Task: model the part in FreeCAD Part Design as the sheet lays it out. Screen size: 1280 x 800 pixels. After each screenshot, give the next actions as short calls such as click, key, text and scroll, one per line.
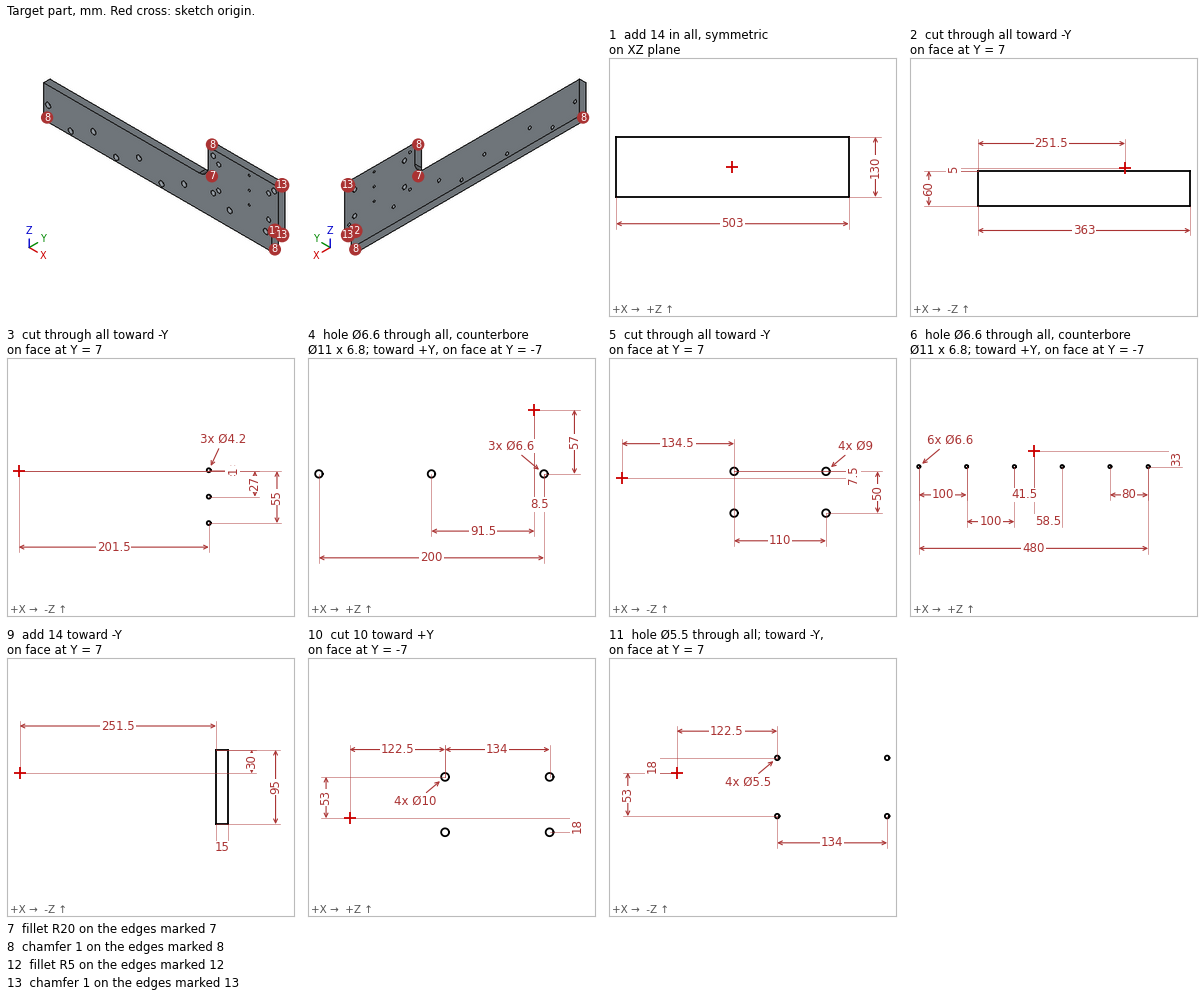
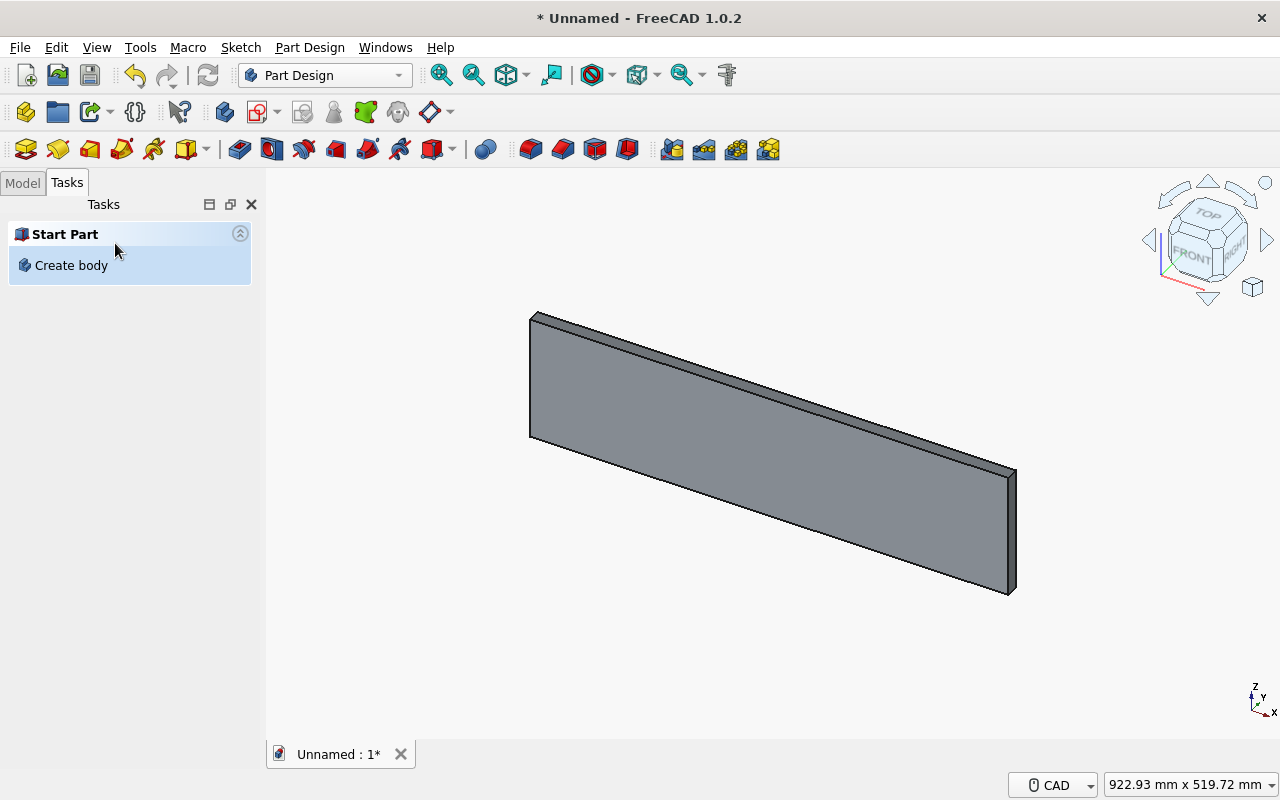
key(4)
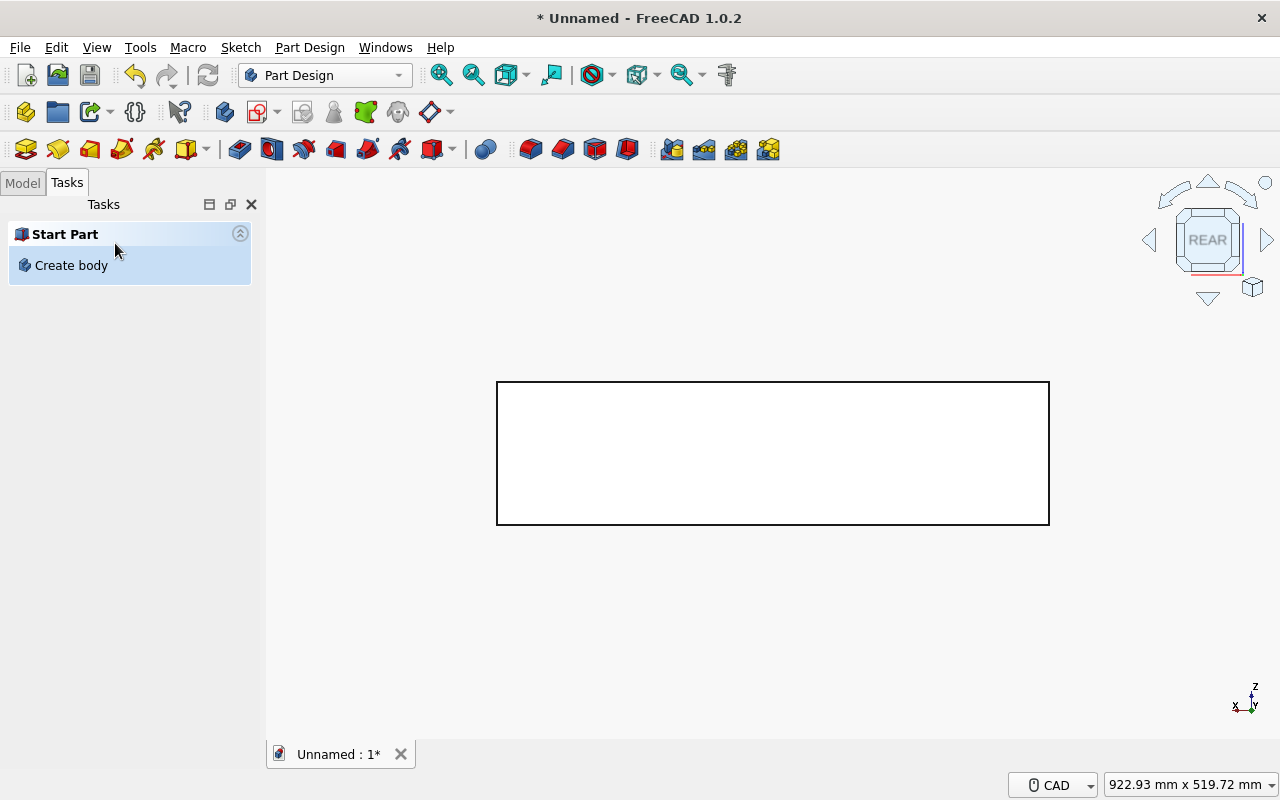
click(615, 452)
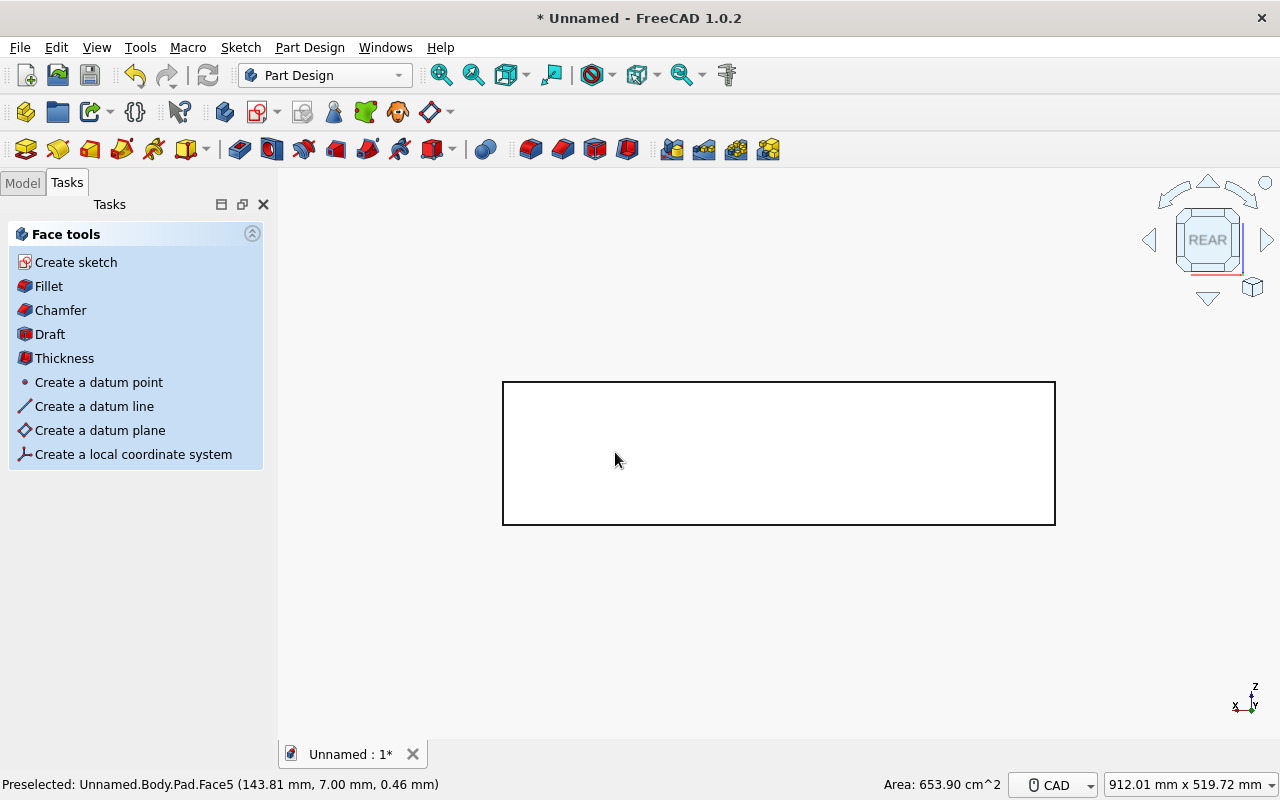
click(258, 112)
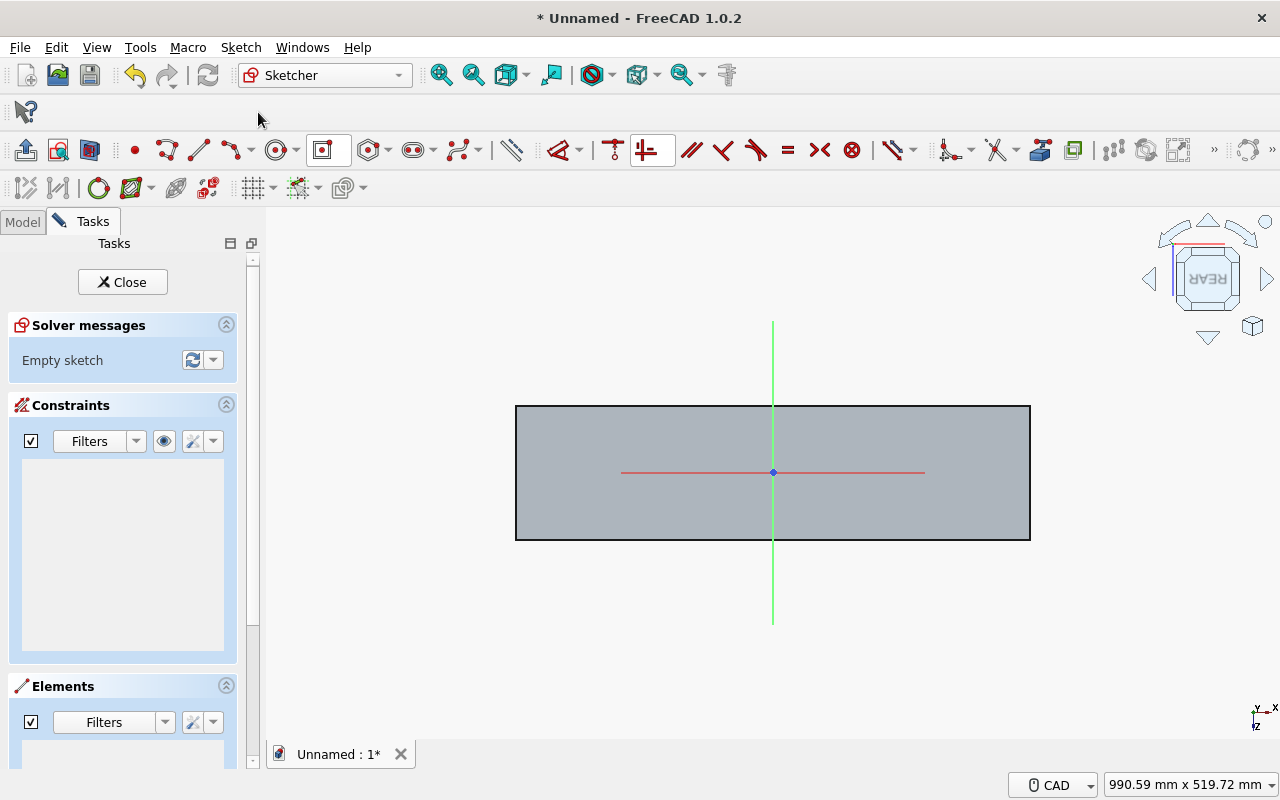
scroll(695, 574, up, 2)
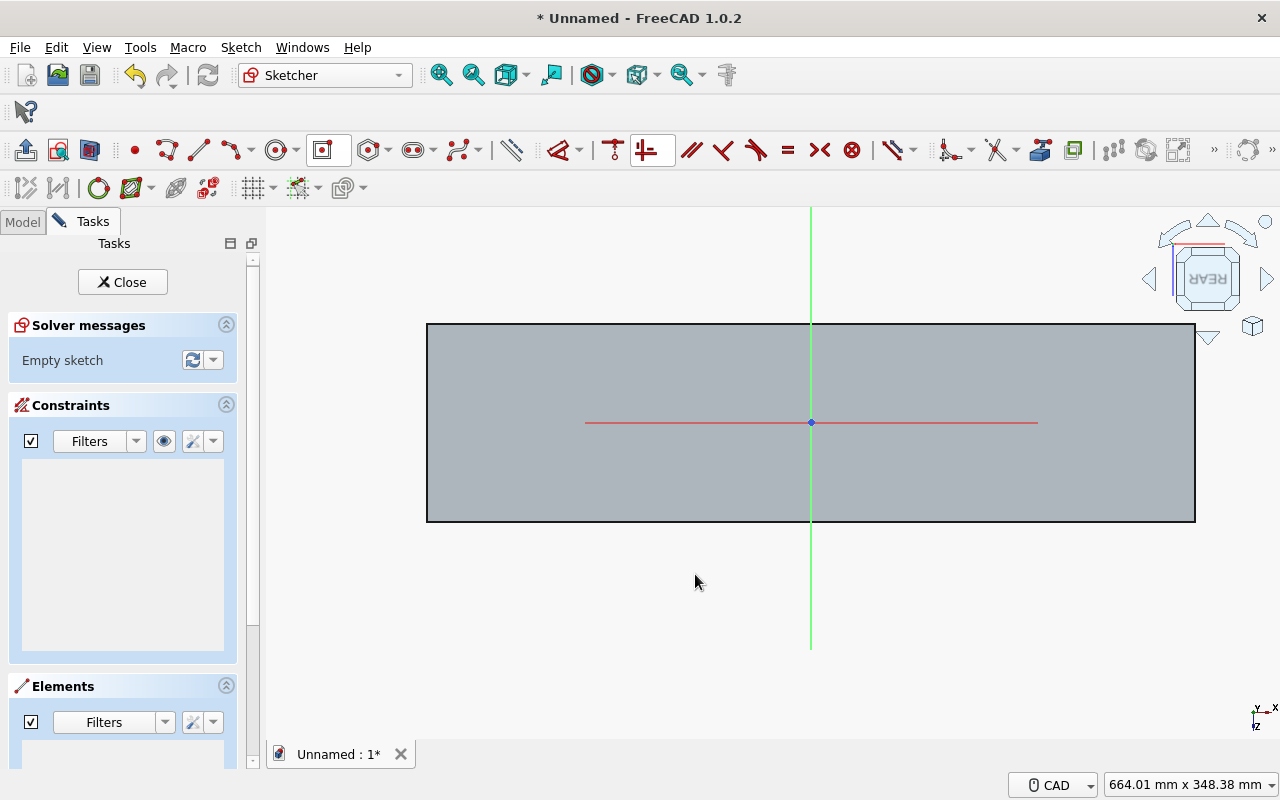
key(g)
key(r)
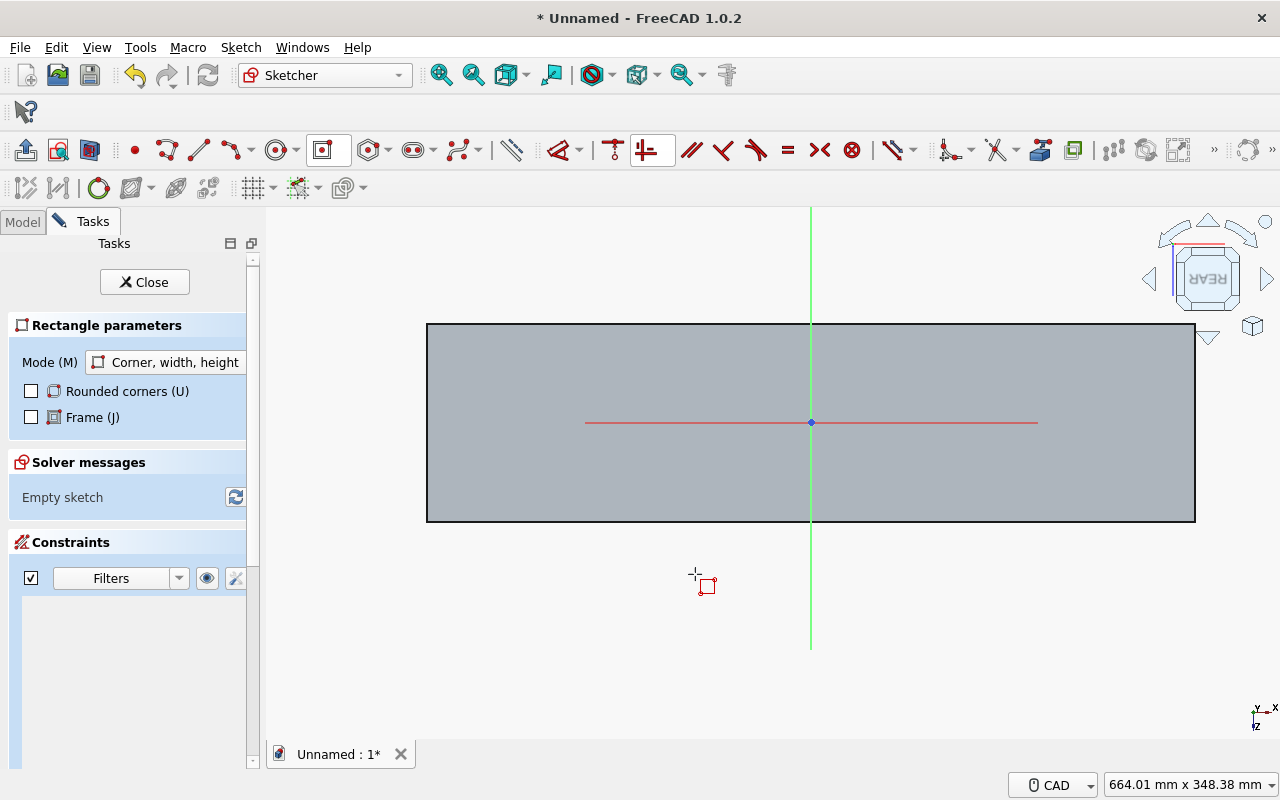
scroll(427, 431, up, 4)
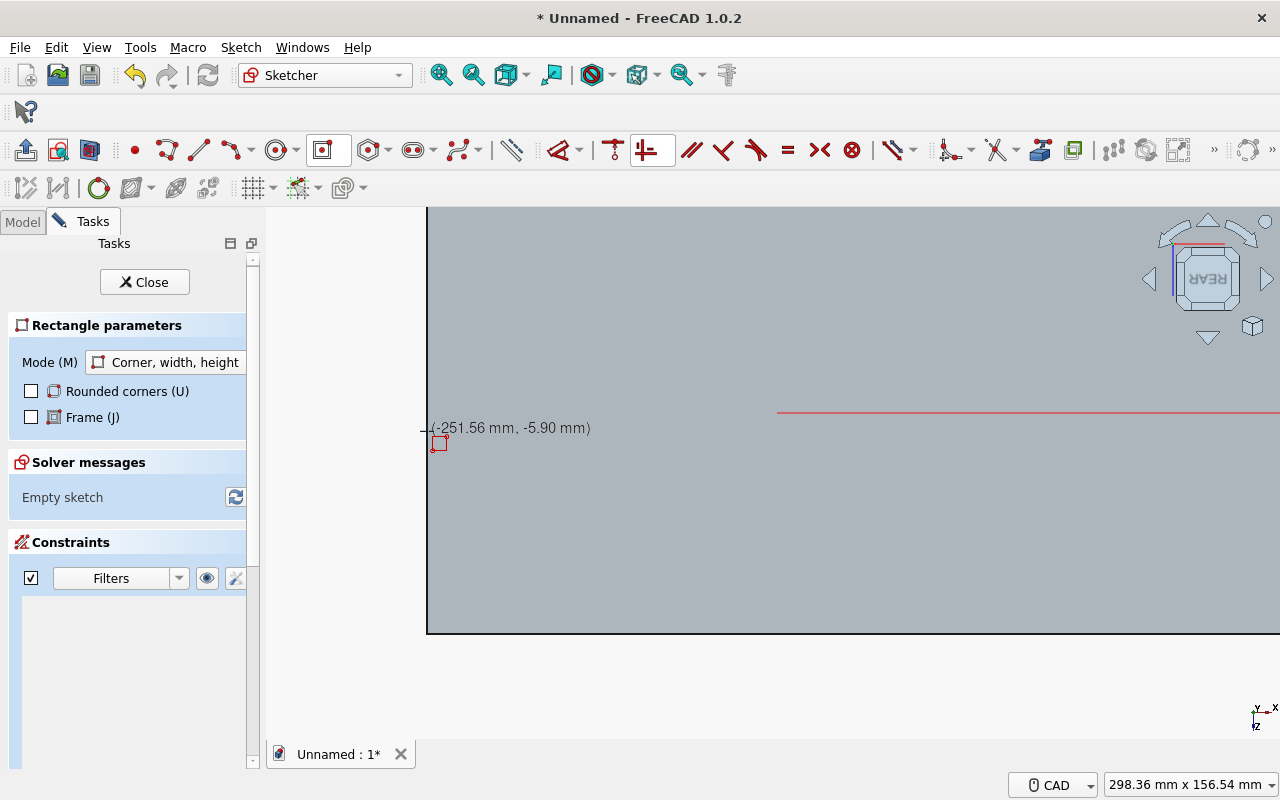
click(427, 430)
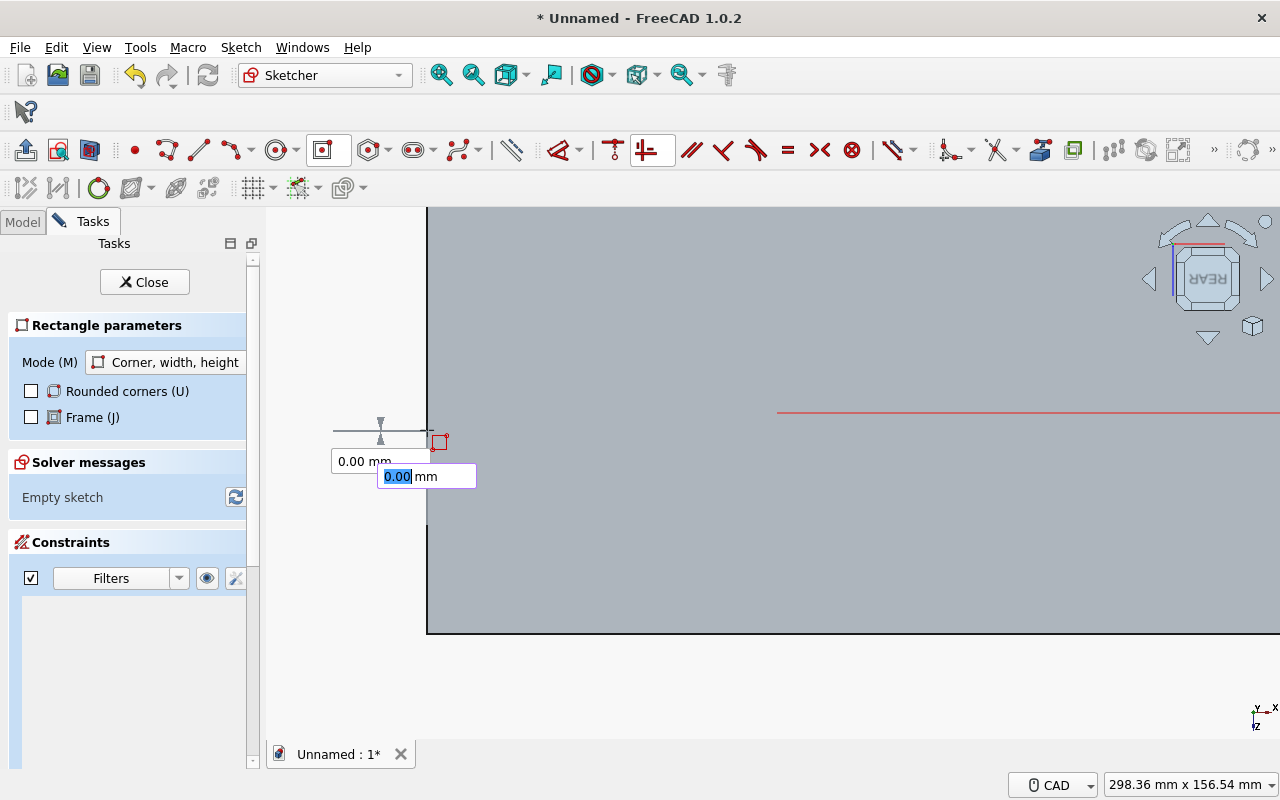
scroll(428, 432, down, 4)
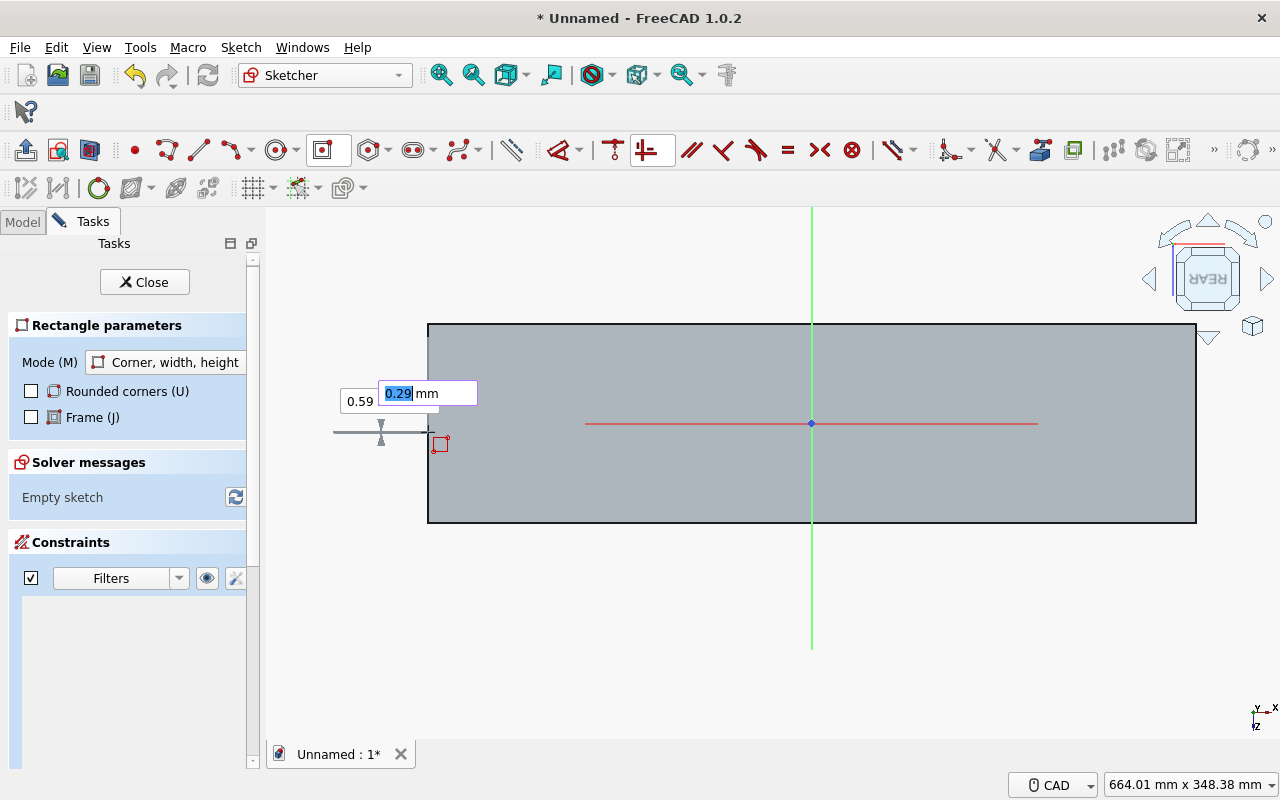
click(982, 523)
key(Escape)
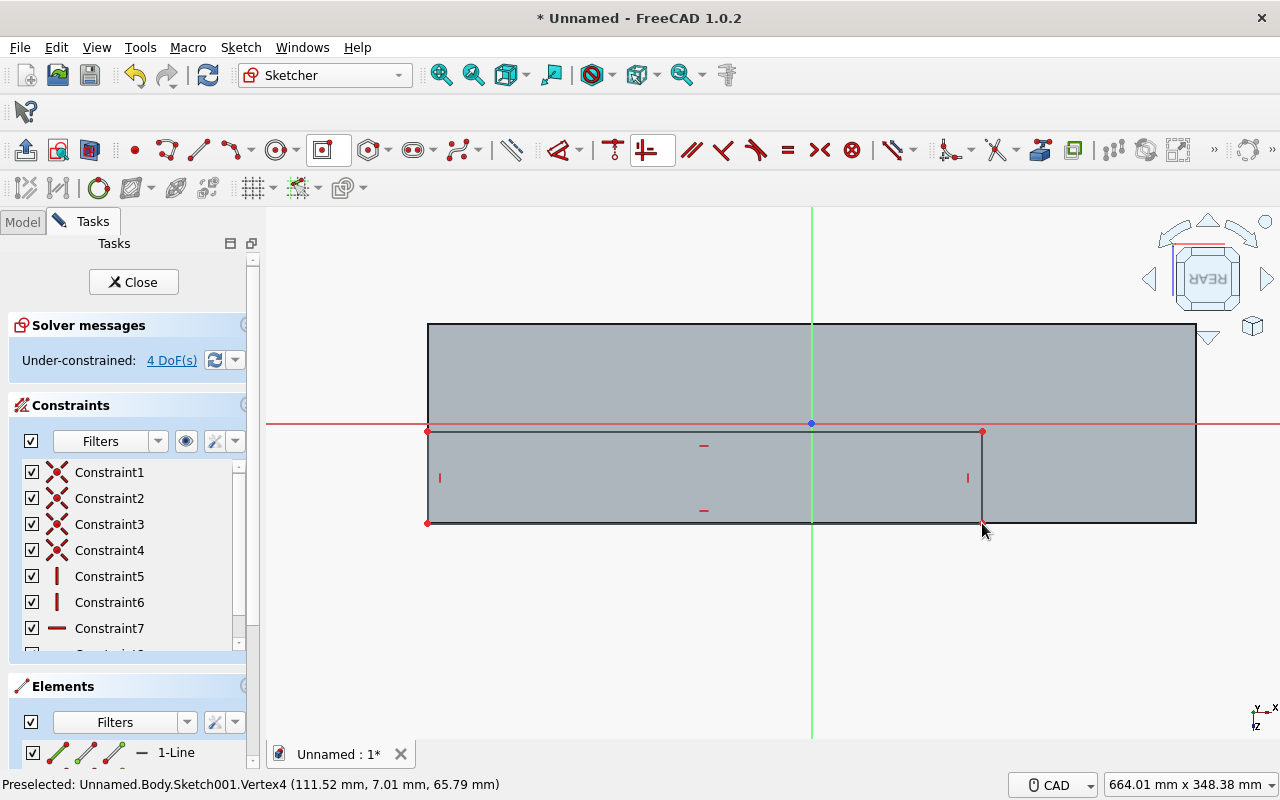
click(428, 459)